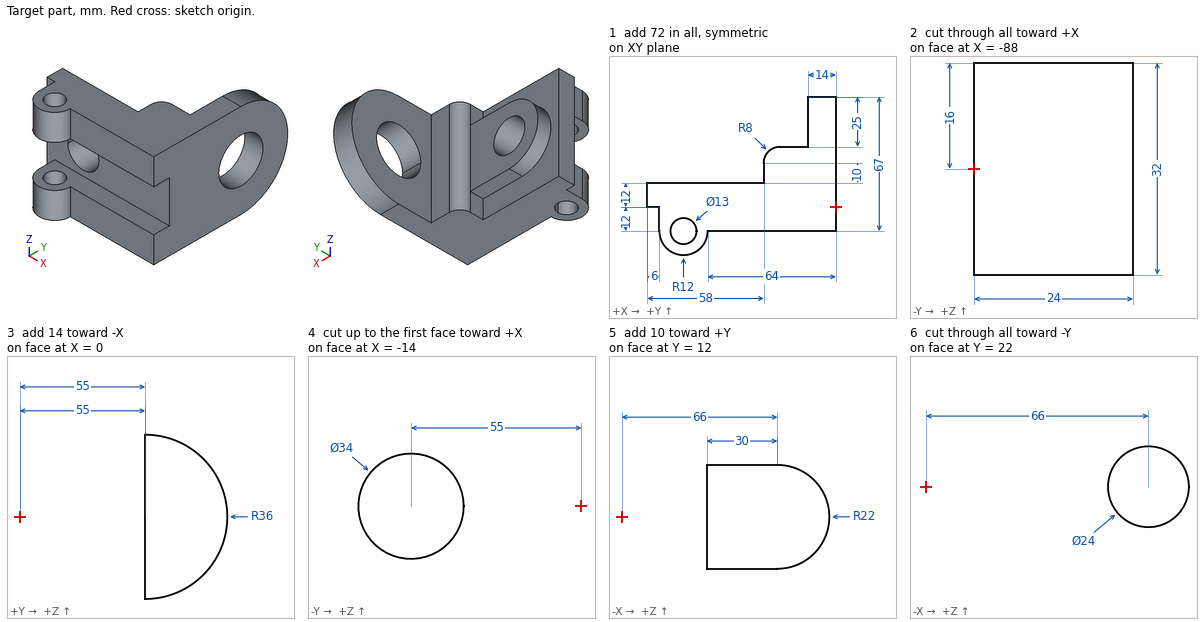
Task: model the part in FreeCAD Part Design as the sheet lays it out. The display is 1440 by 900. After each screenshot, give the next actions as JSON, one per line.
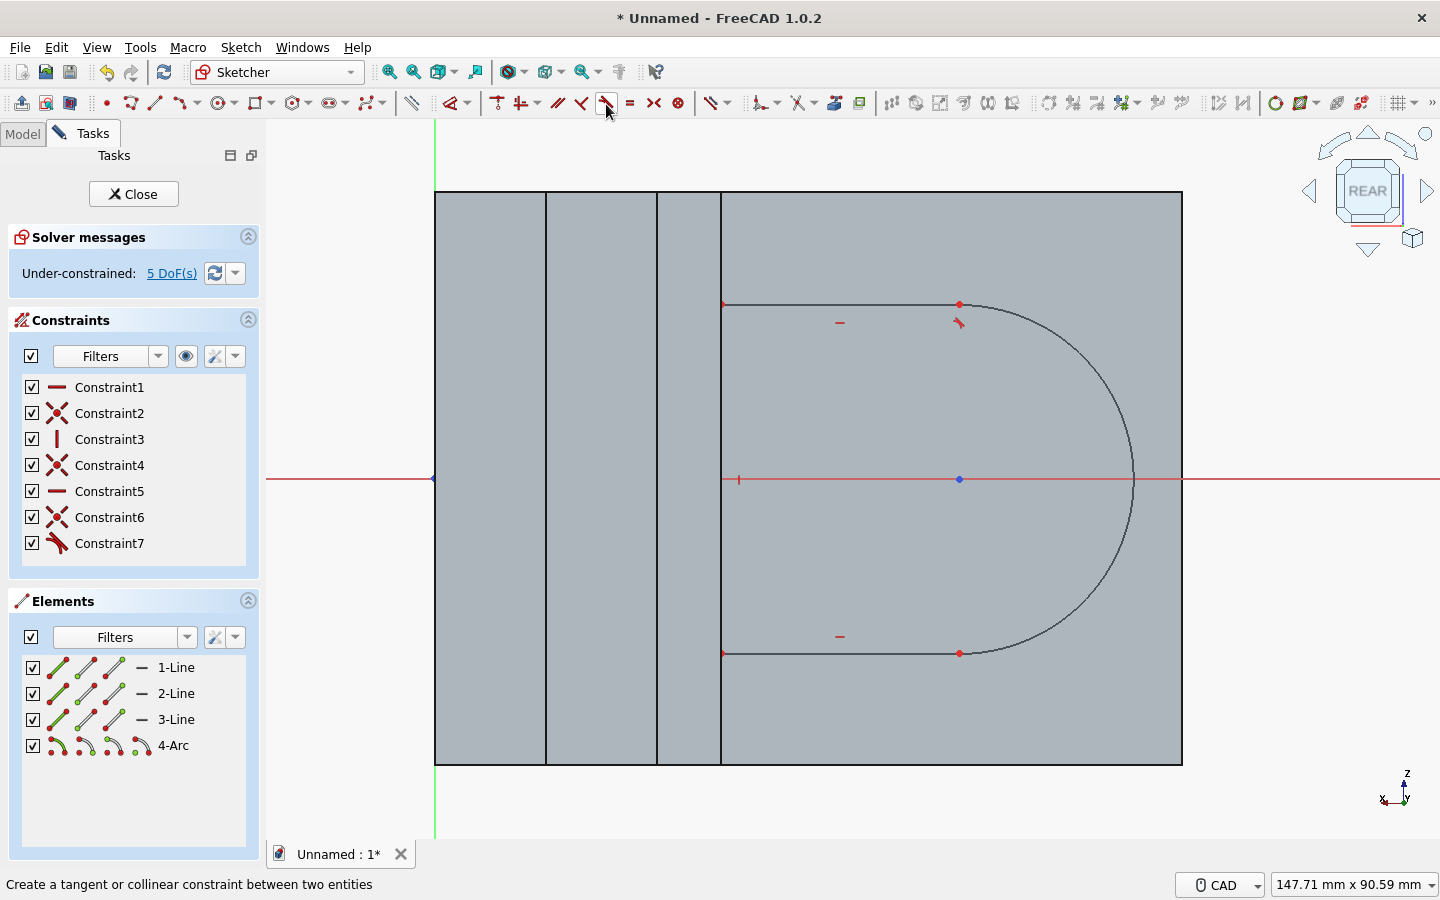
{"action": "left_click", "coordinate": [792, 654]}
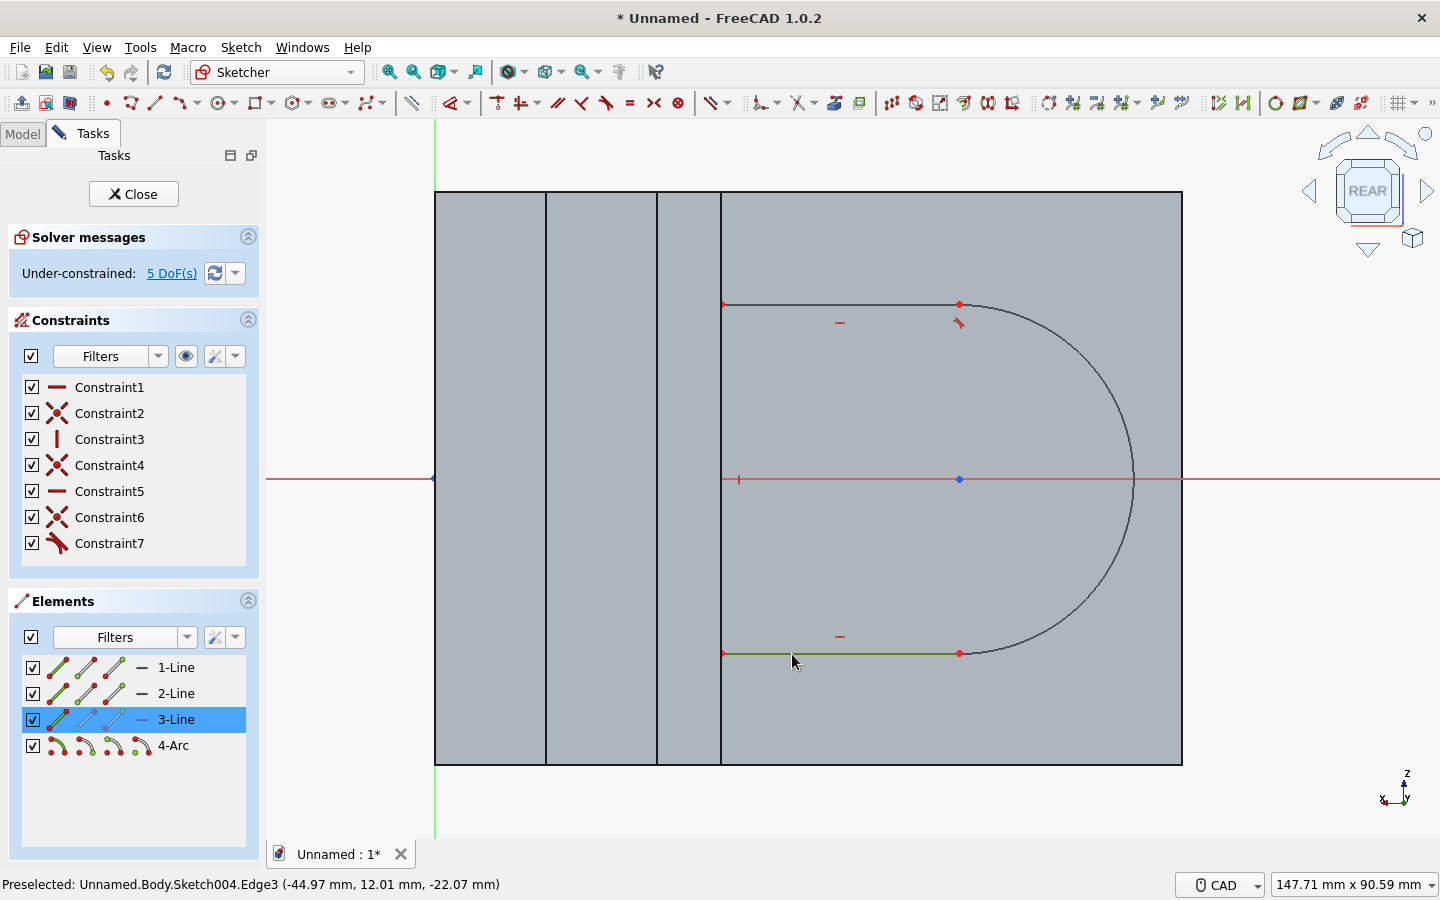
{"action": "left_click", "coordinate": [1100, 582]}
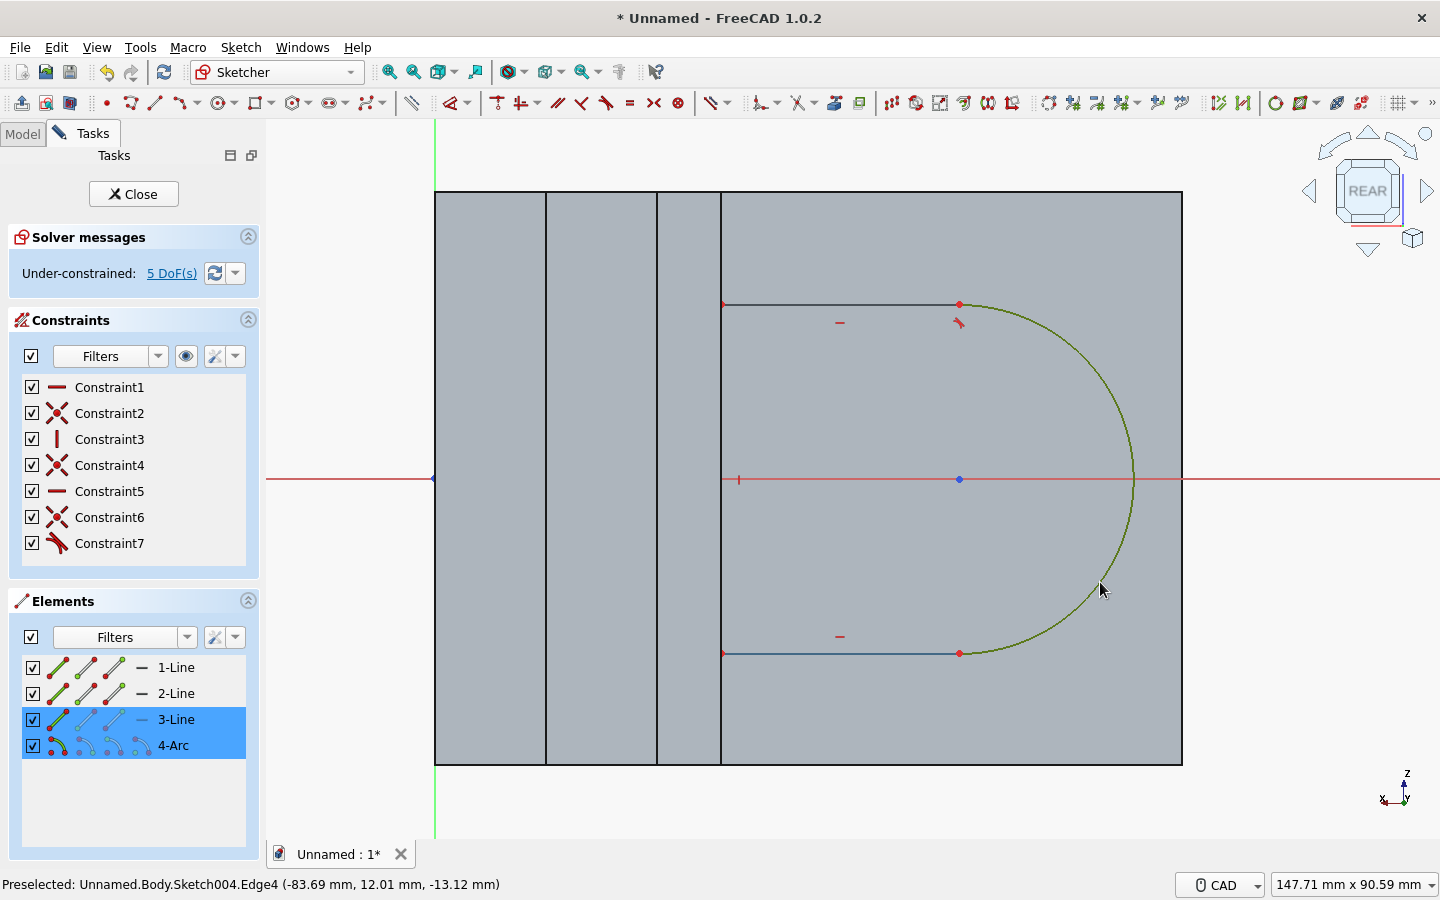
{"action": "left_click", "coordinate": [606, 104]}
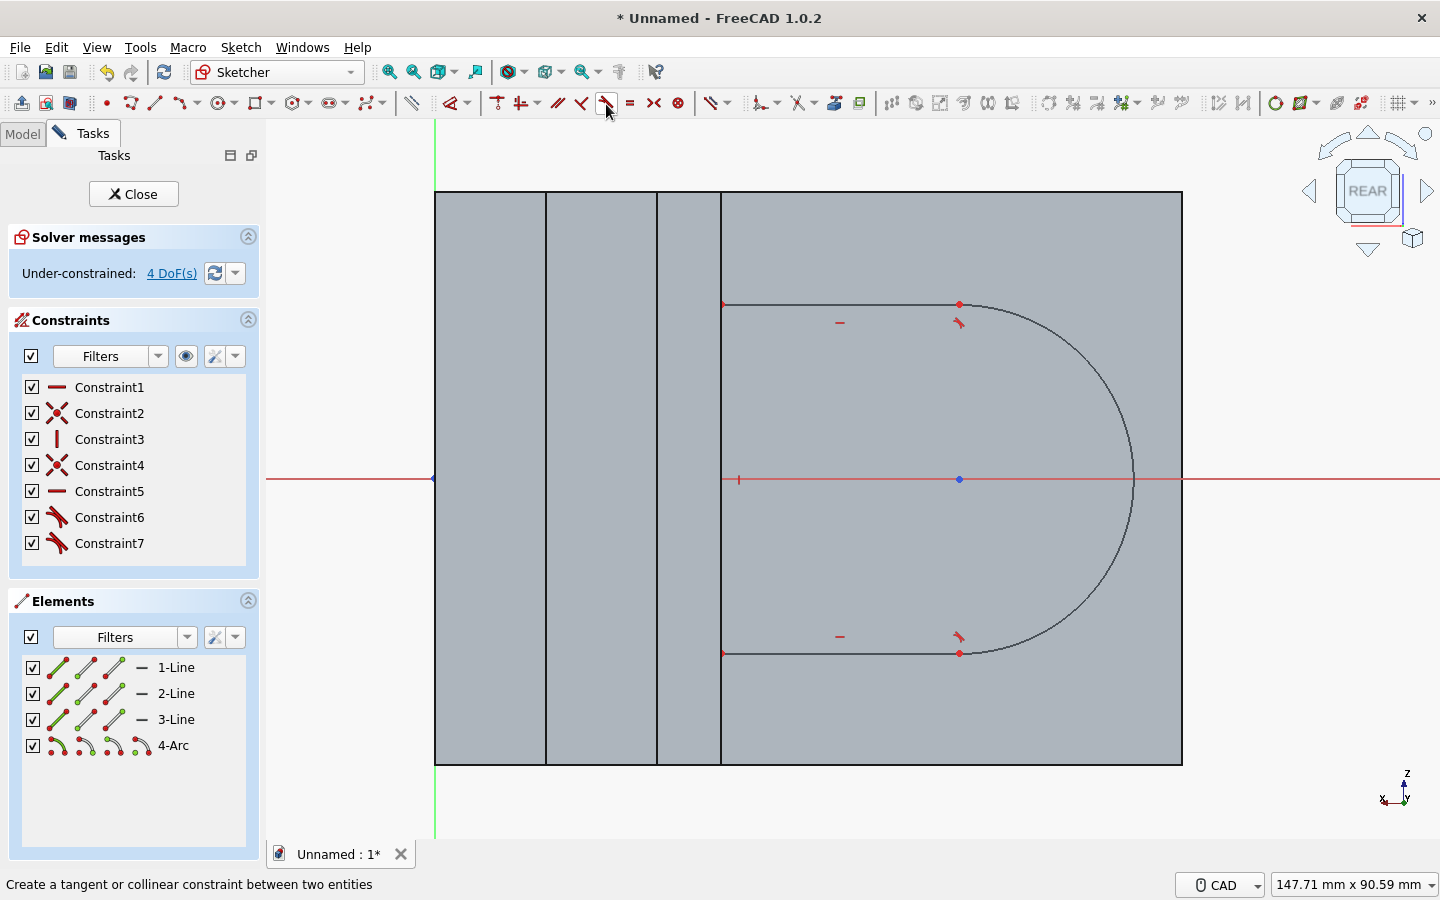
{"action": "left_click", "coordinate": [959, 479]}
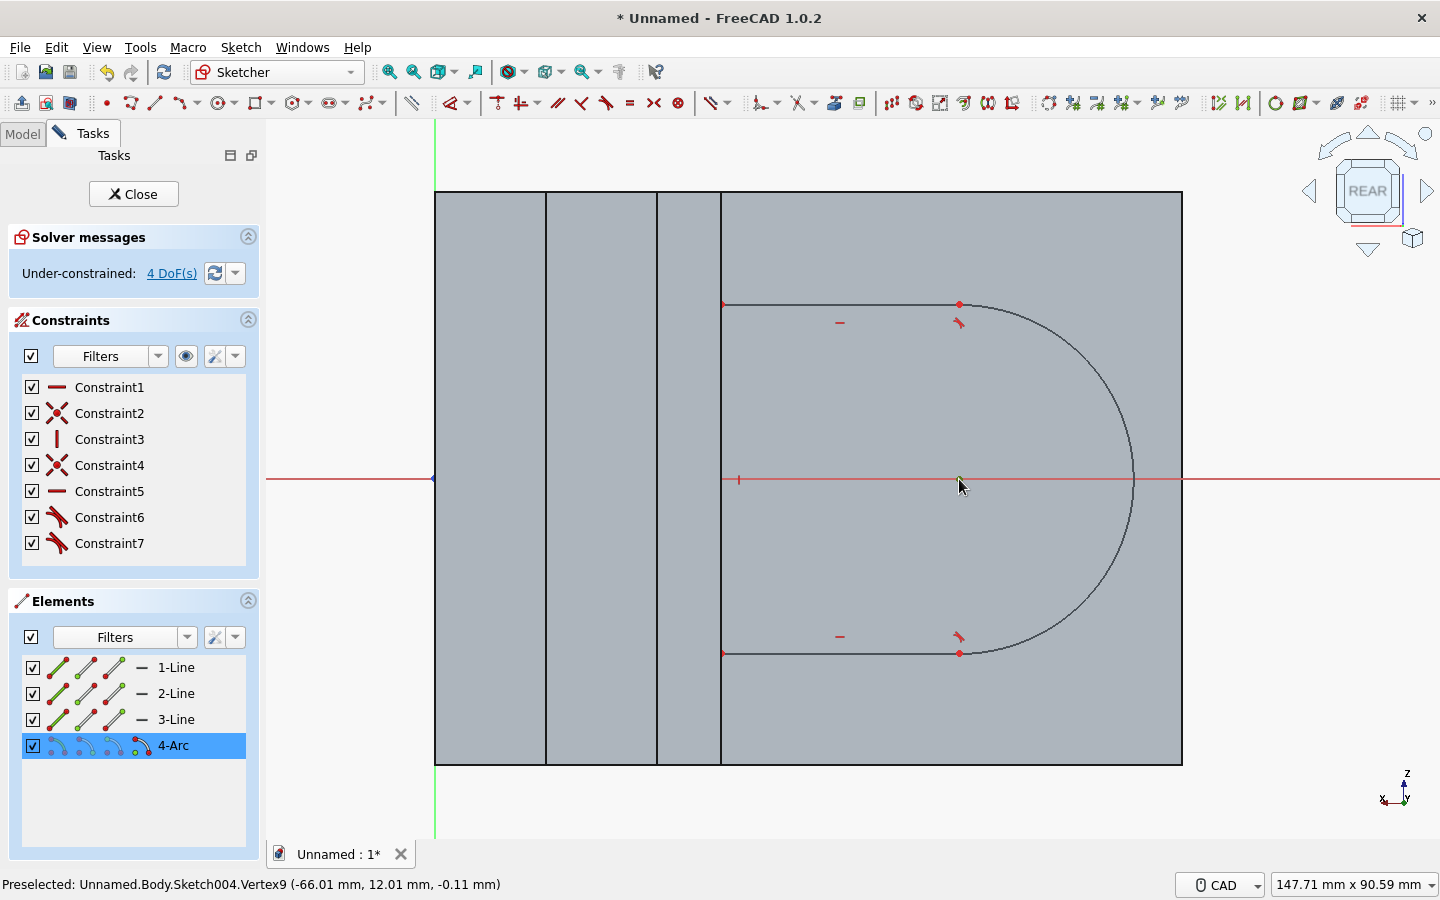
{"action": "left_click", "coordinate": [364, 479]}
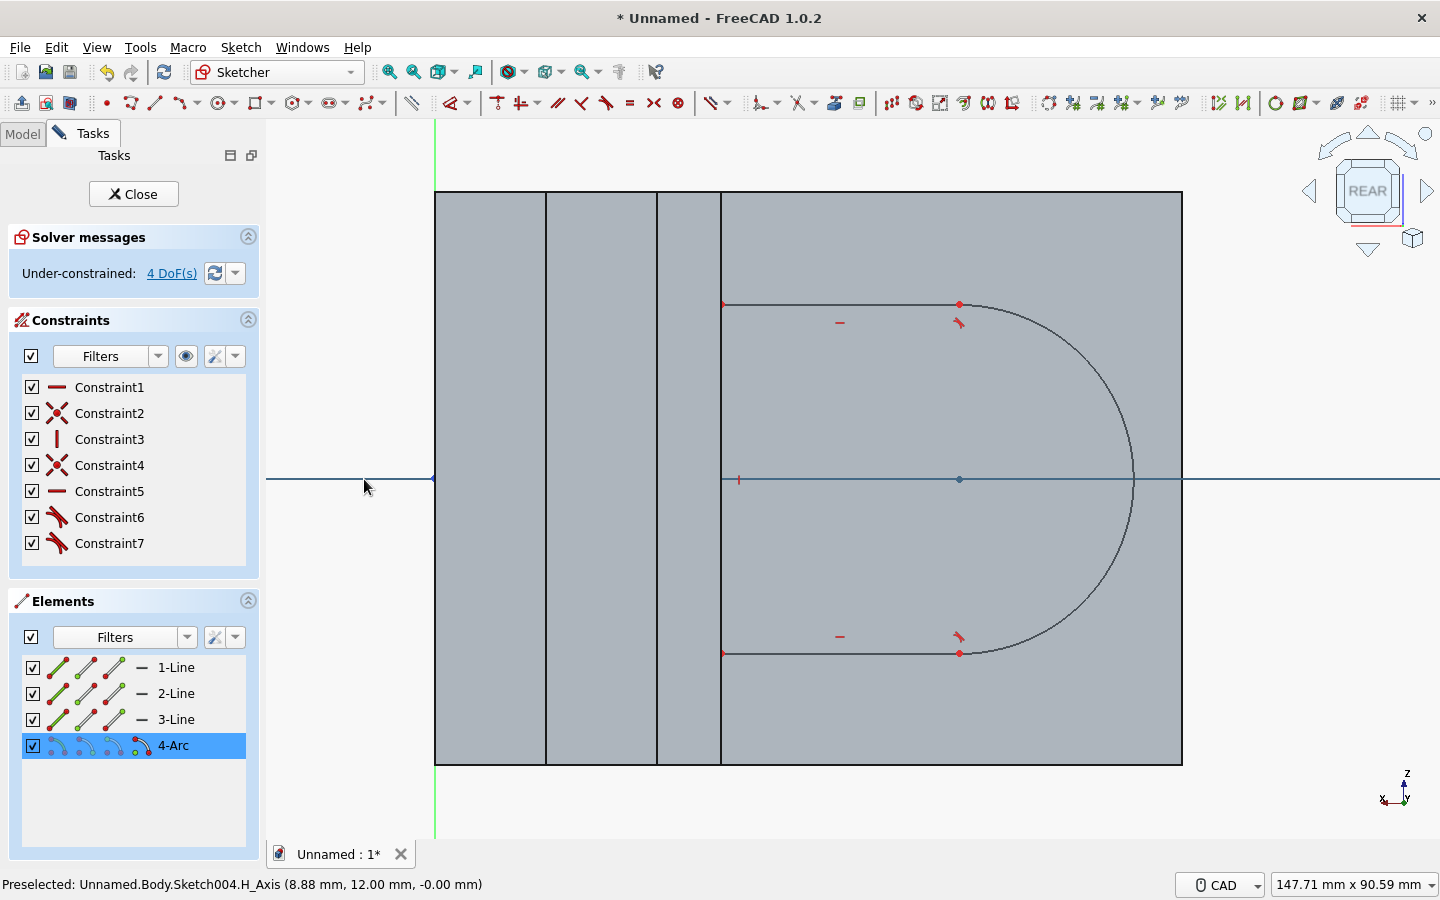
{"action": "left_click", "coordinate": [498, 104]}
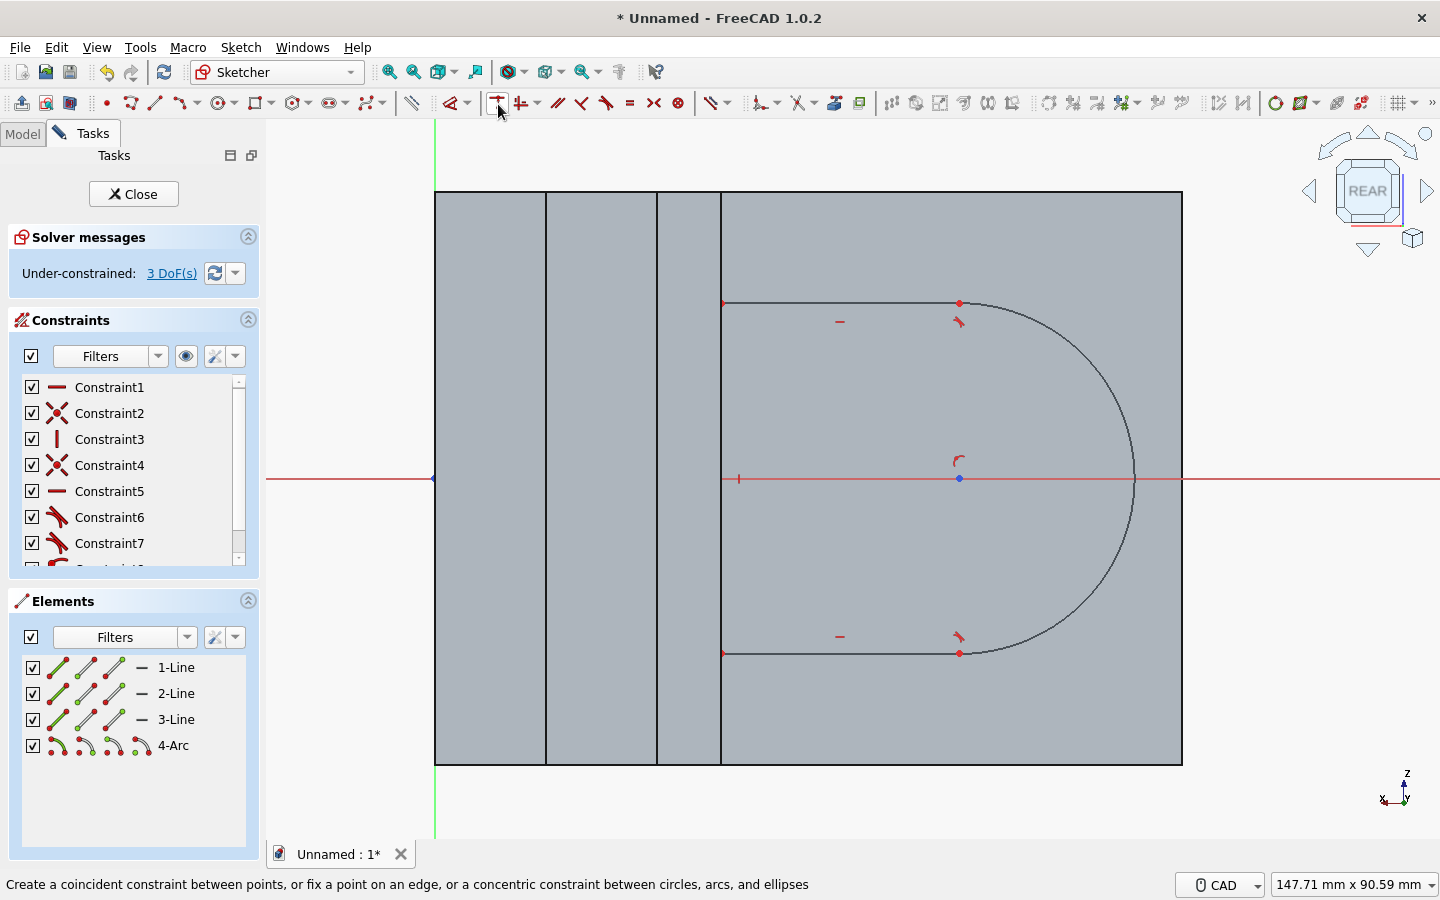
{"action": "left_click", "coordinate": [450, 104]}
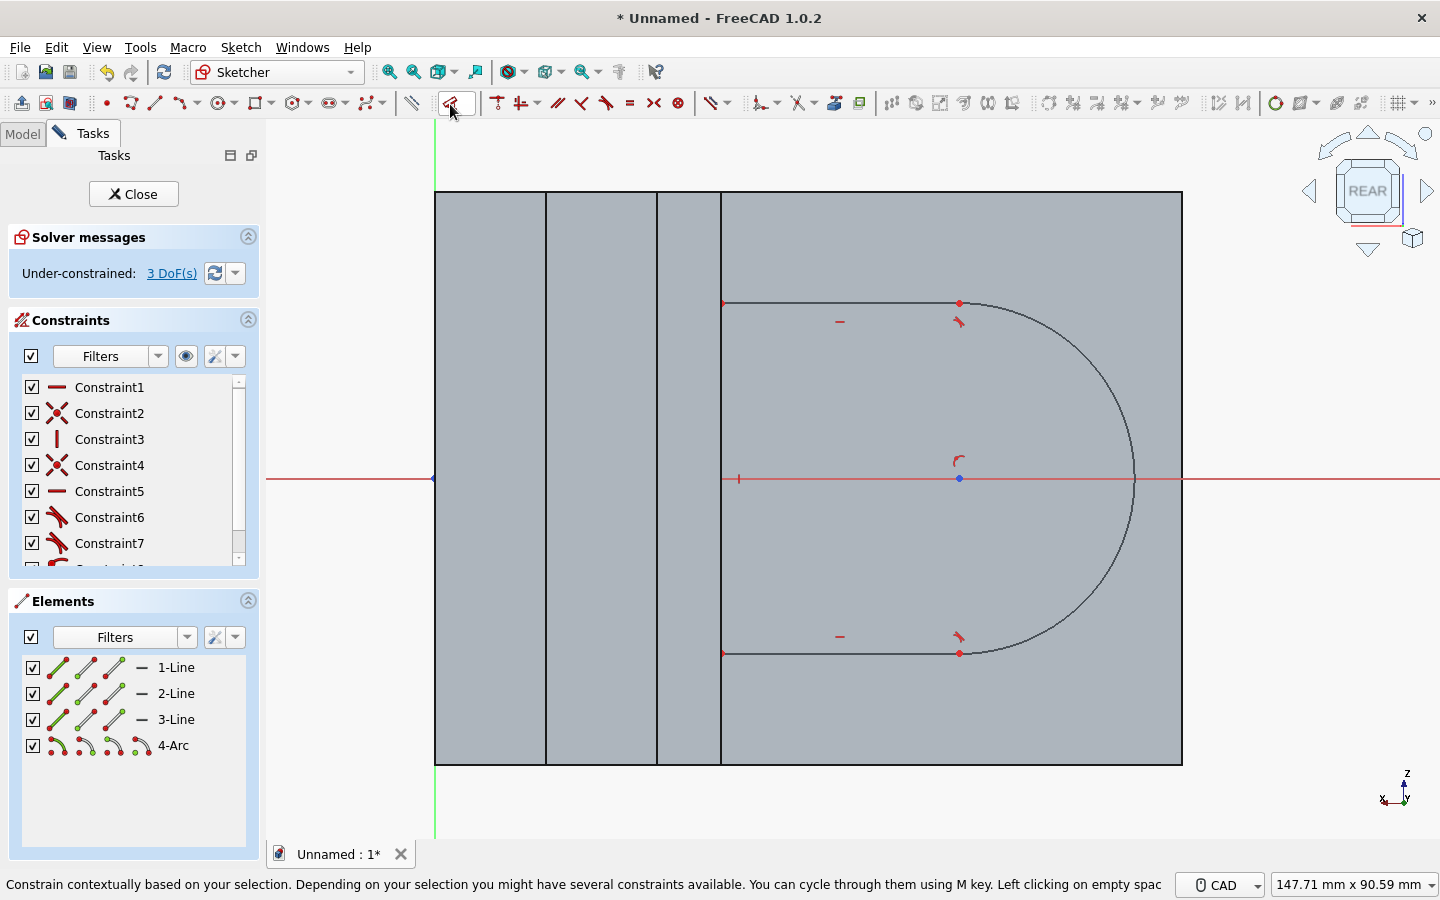
{"action": "left_click", "coordinate": [1101, 582]}
{"action": "left_click", "coordinate": [1127, 601]}